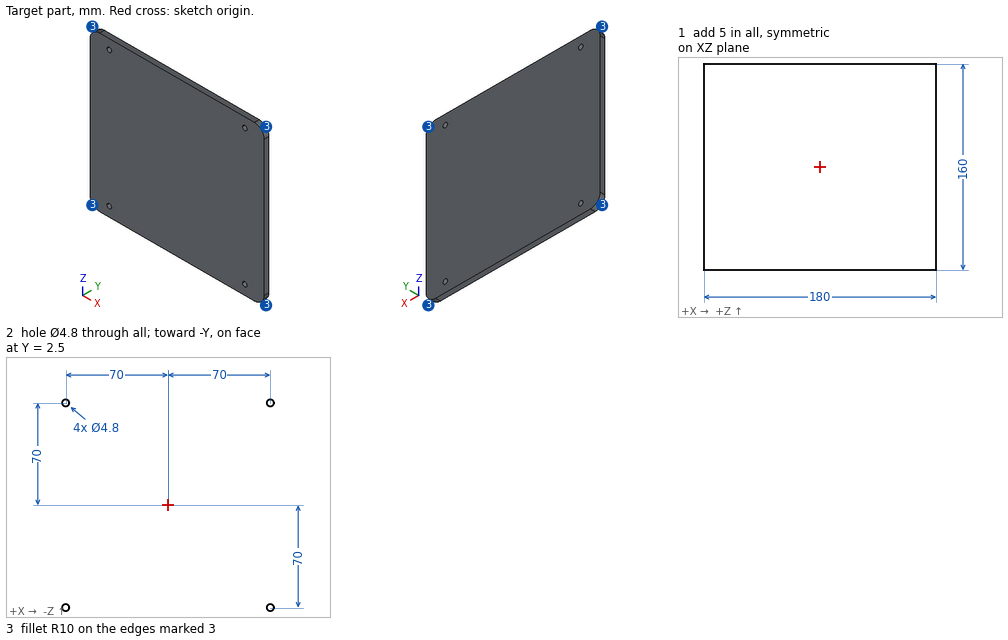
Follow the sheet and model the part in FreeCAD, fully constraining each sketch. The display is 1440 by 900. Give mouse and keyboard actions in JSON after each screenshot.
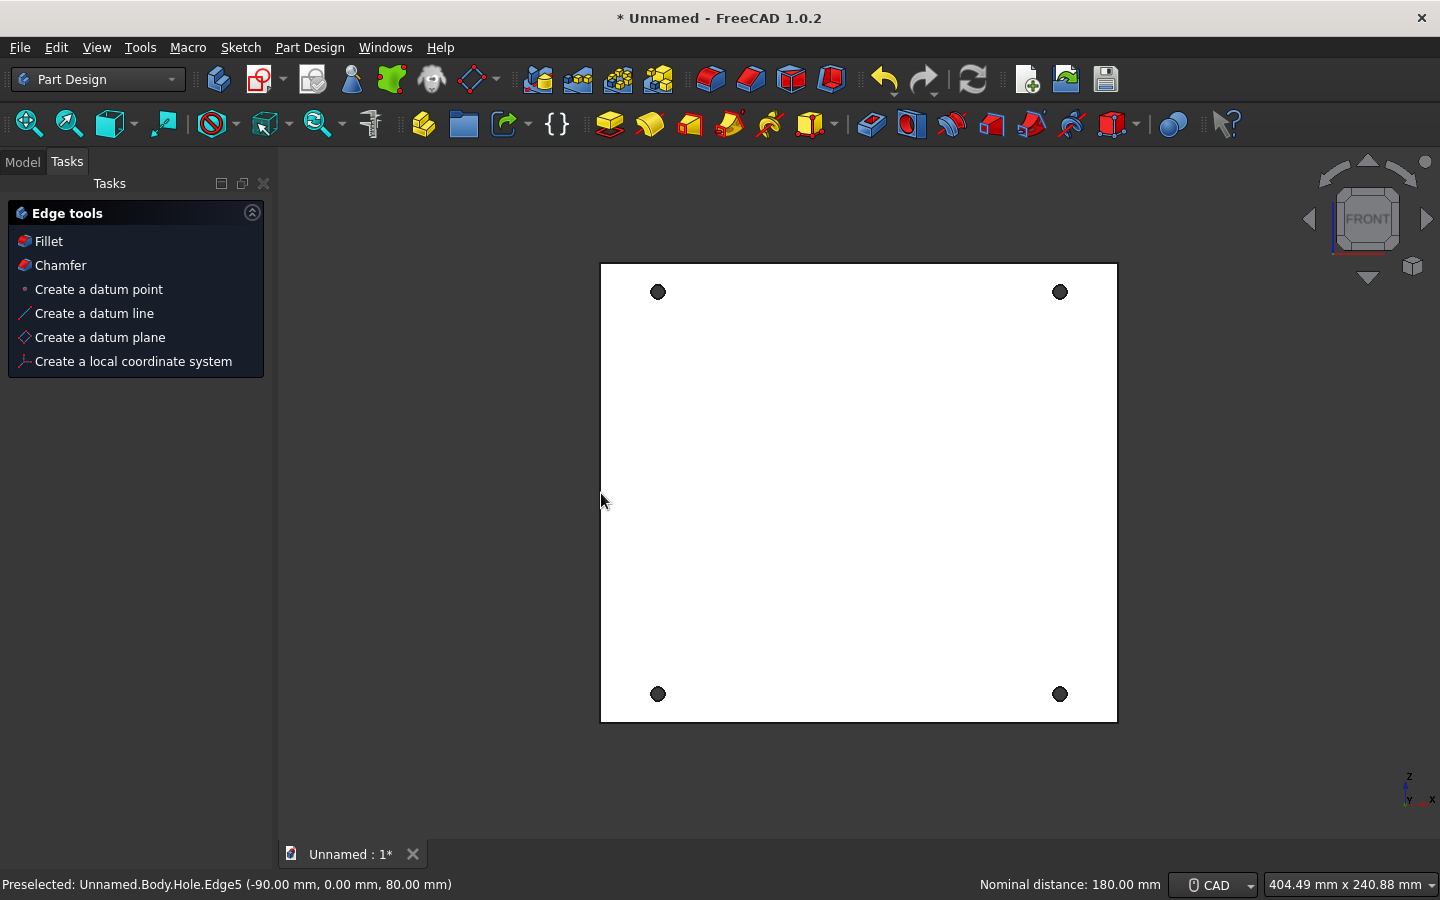
{"action": "scroll", "coordinate": [600, 722], "scroll_direction": "up", "scroll_amount": 6}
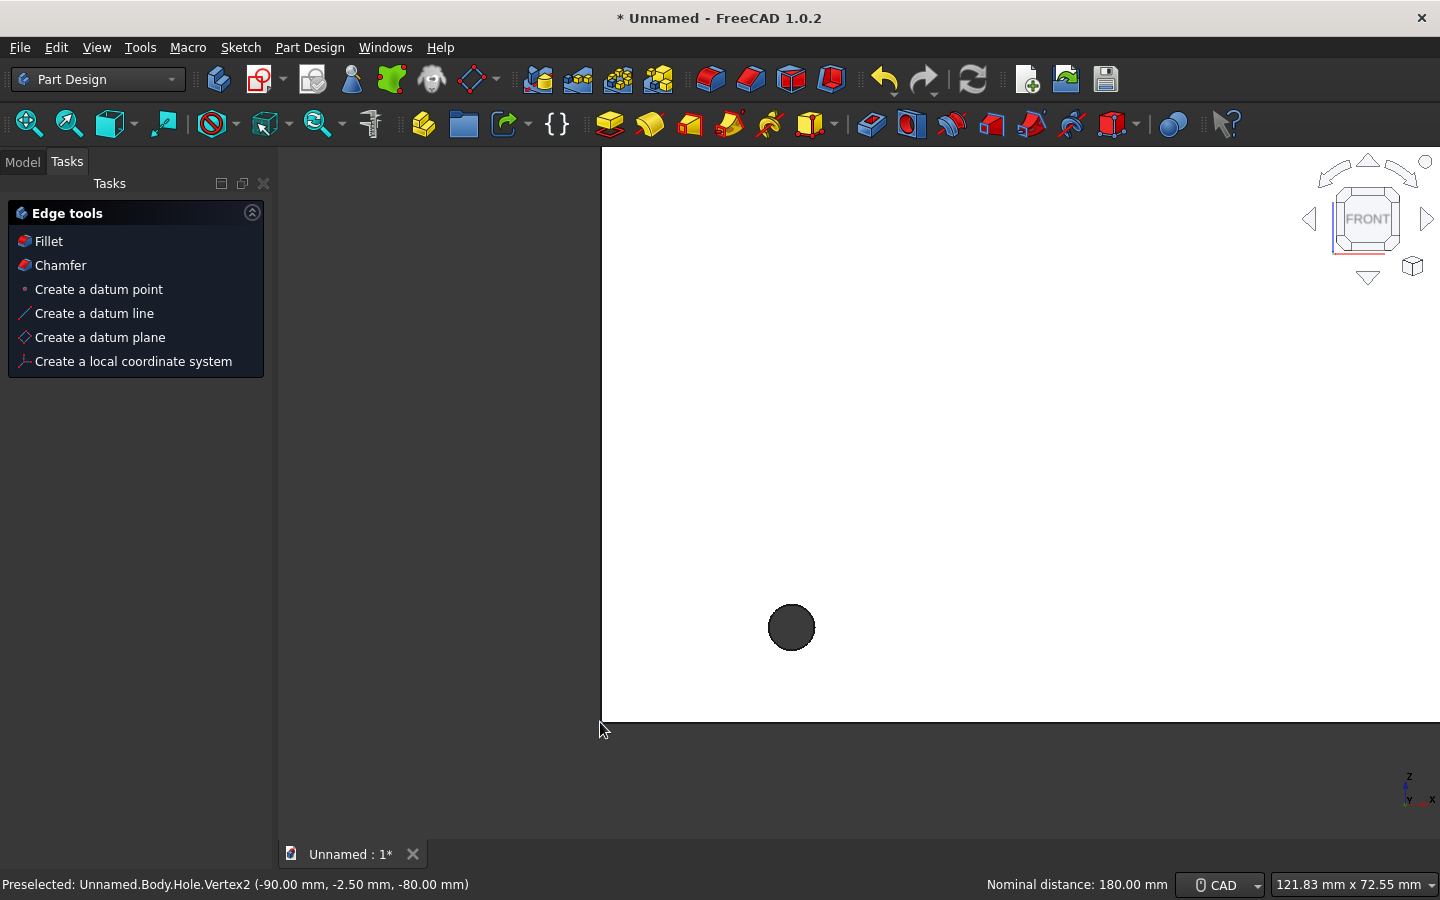
{"action": "left_click", "coordinate": [30, 124]}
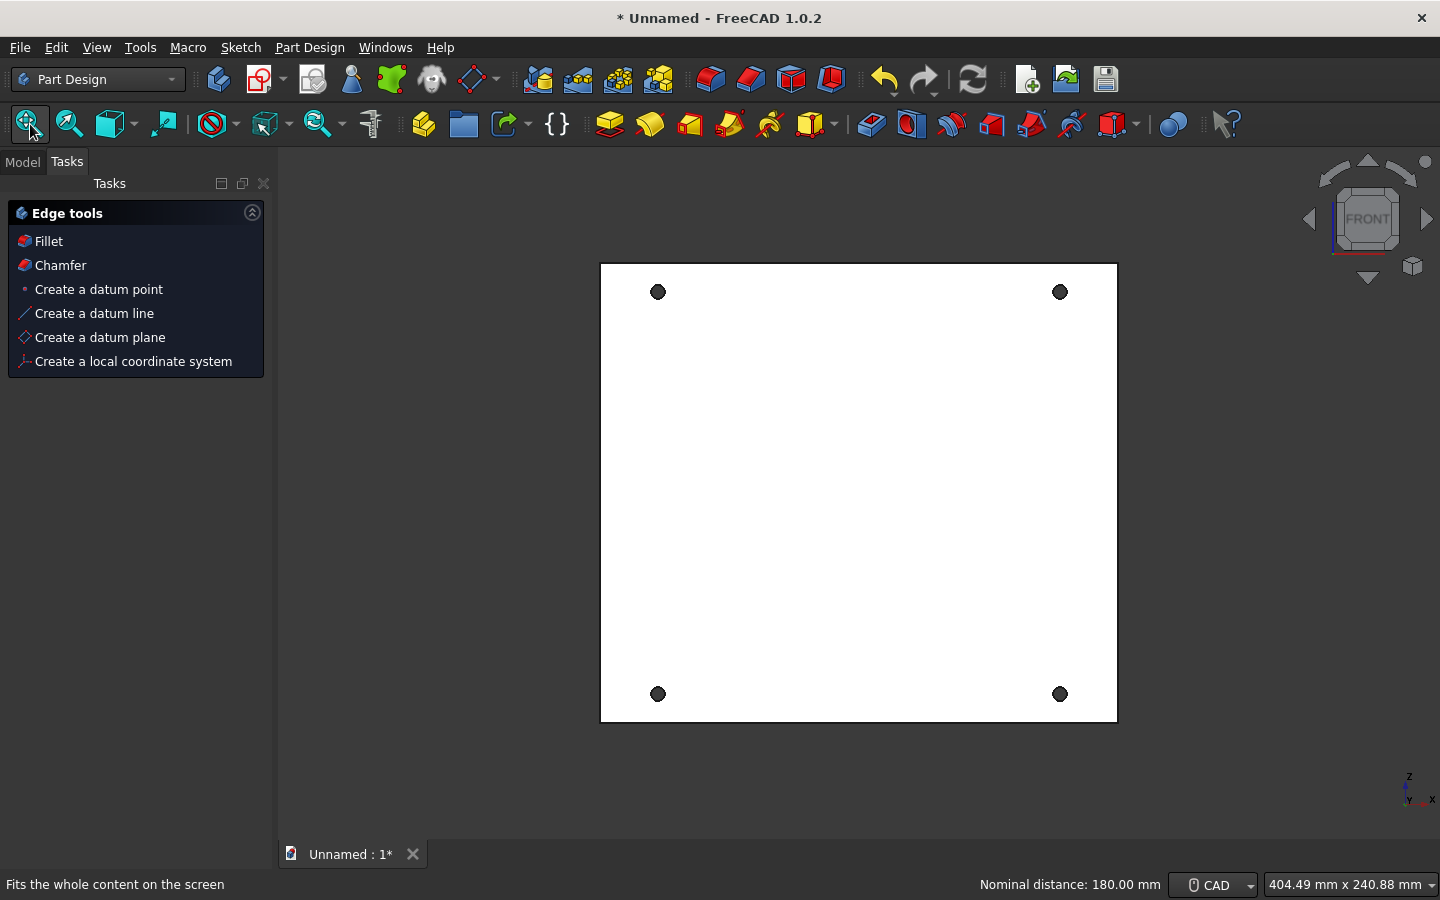
{"action": "key", "text": "3"}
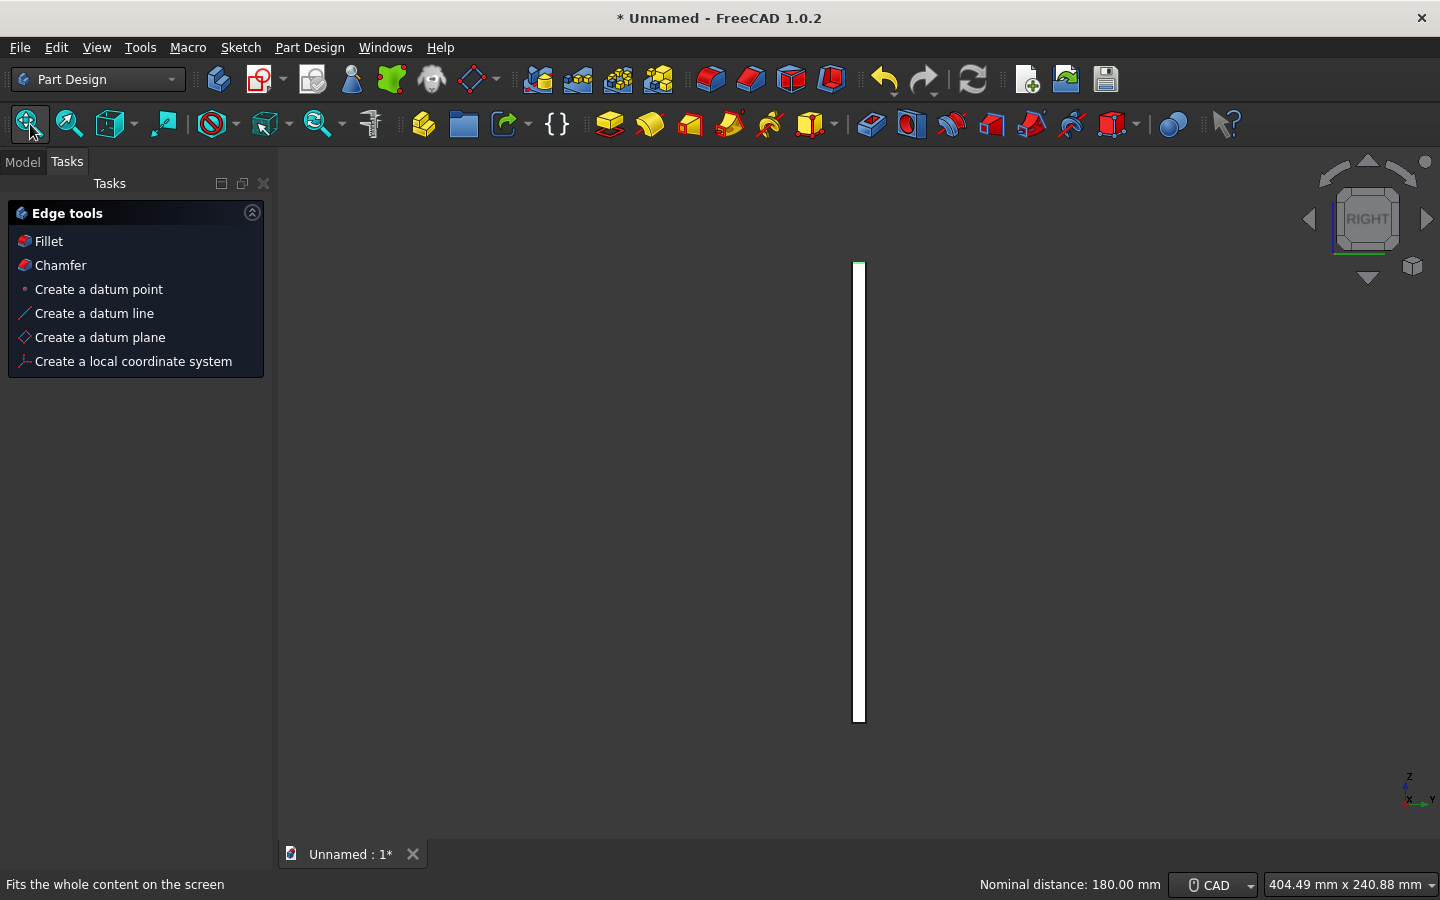
{"action": "left_click", "coordinate": [859, 722], "text": "ctrl"}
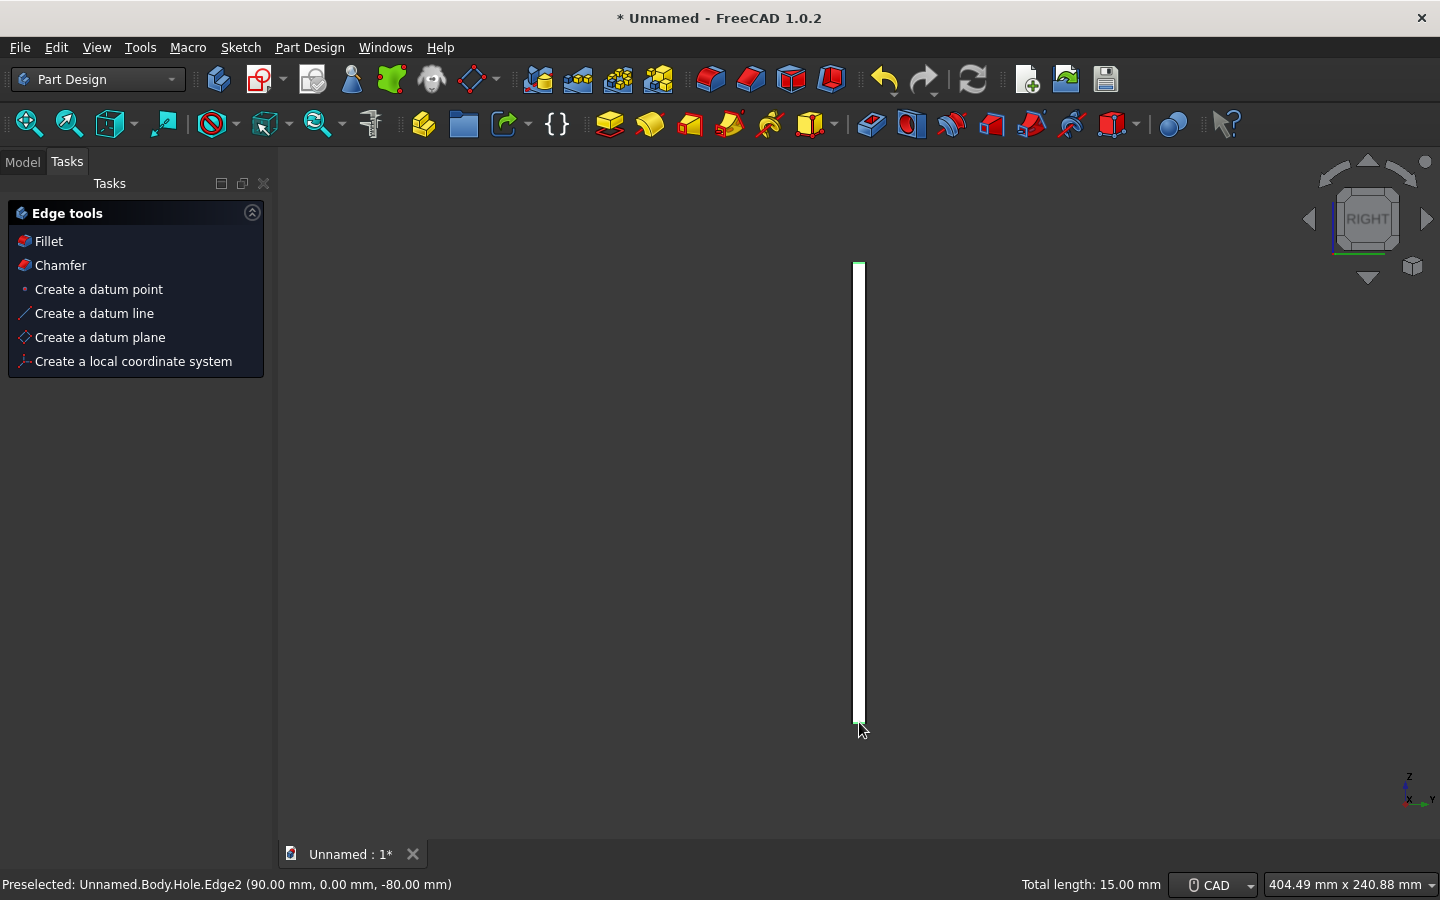
{"action": "scroll", "coordinate": [859, 722], "scroll_direction": "up", "scroll_amount": 6}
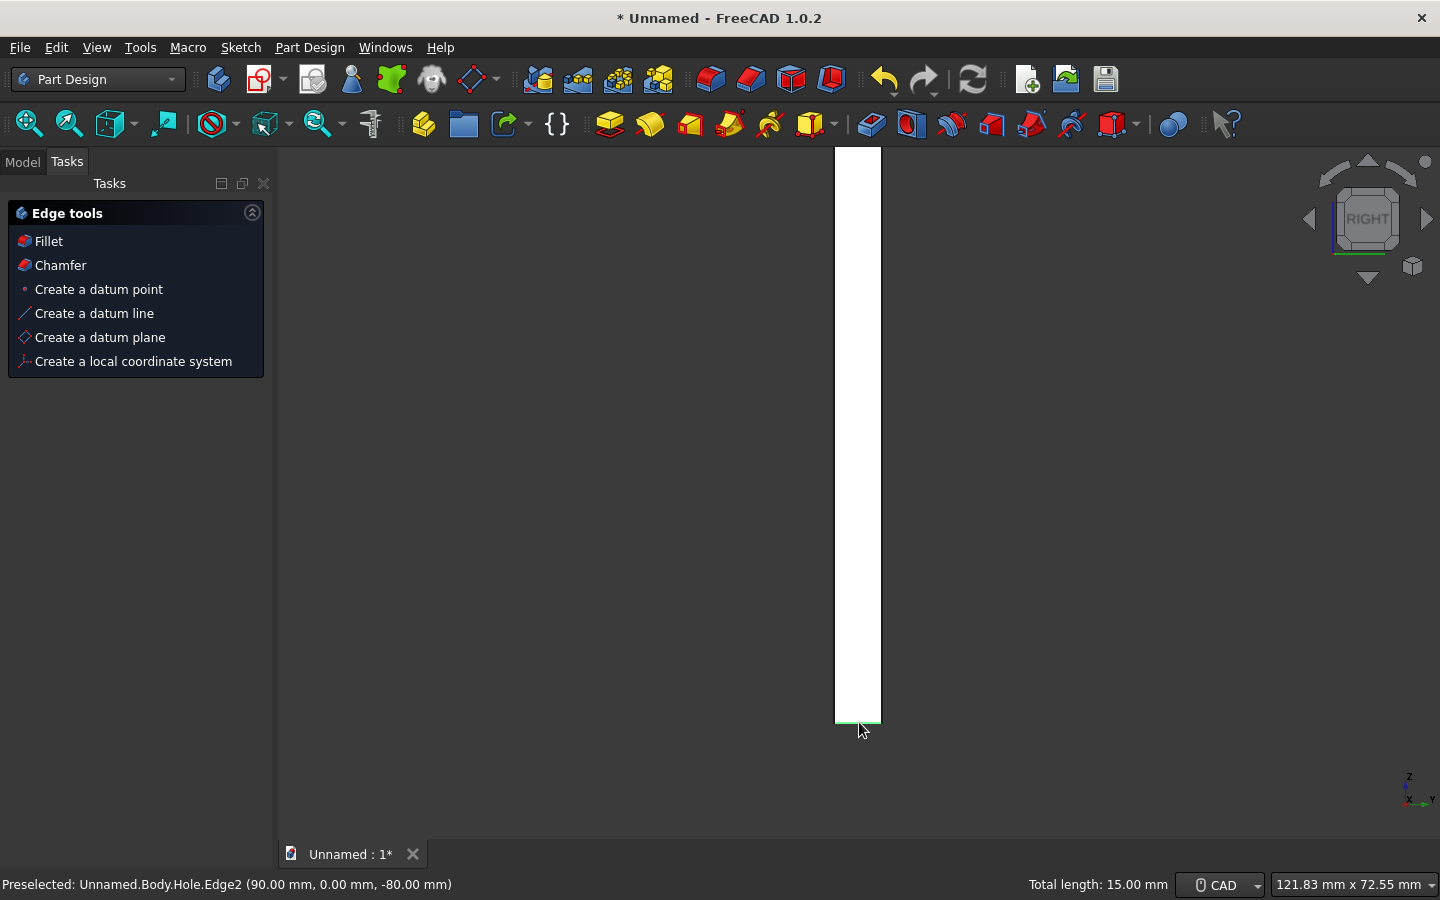
{"action": "left_click", "coordinate": [30, 124]}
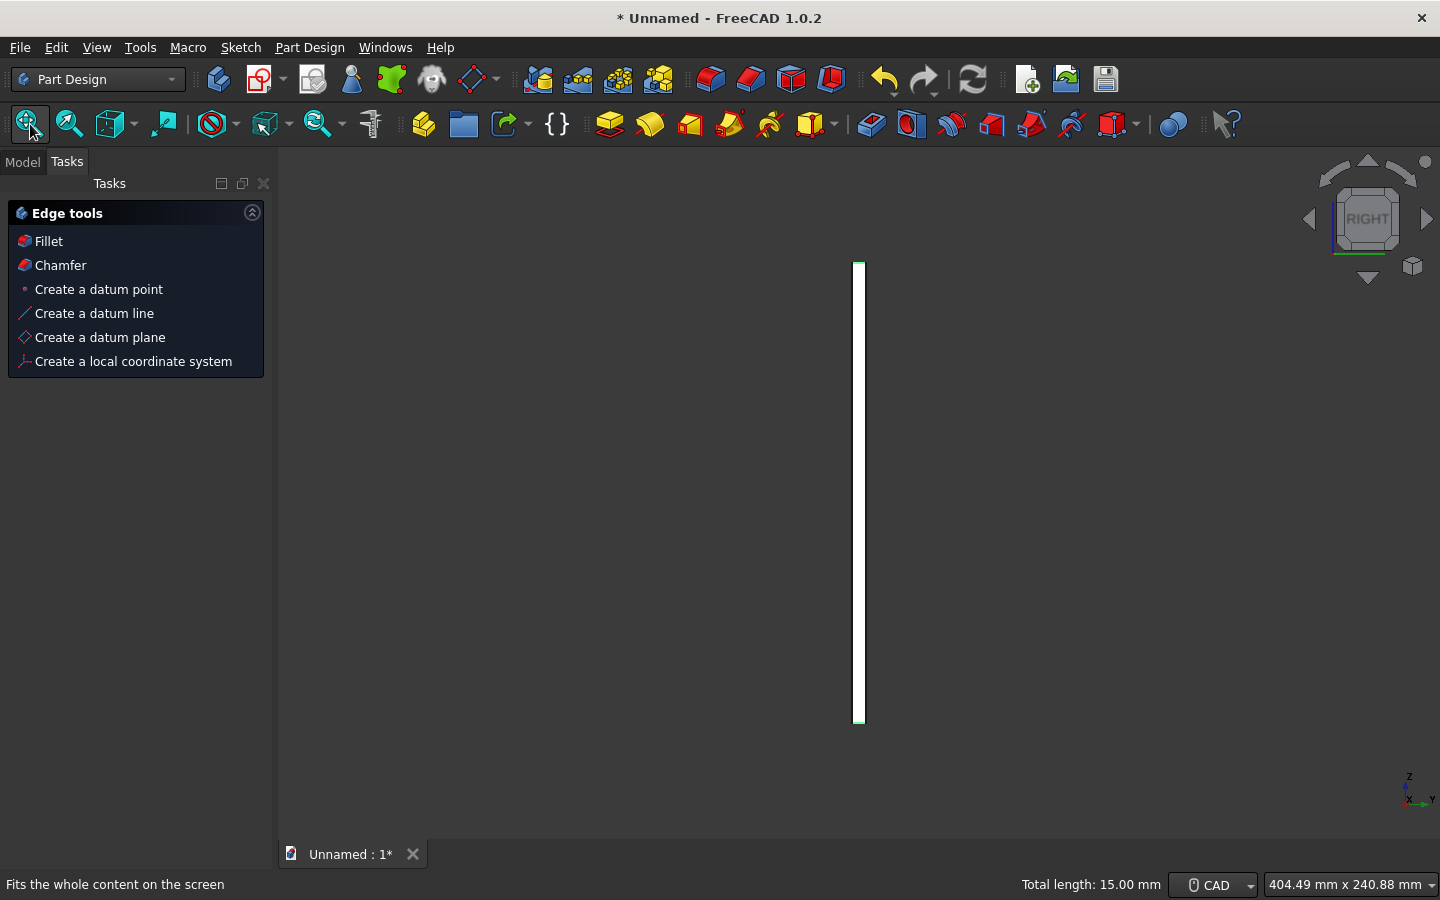
{"action": "key", "text": "5"}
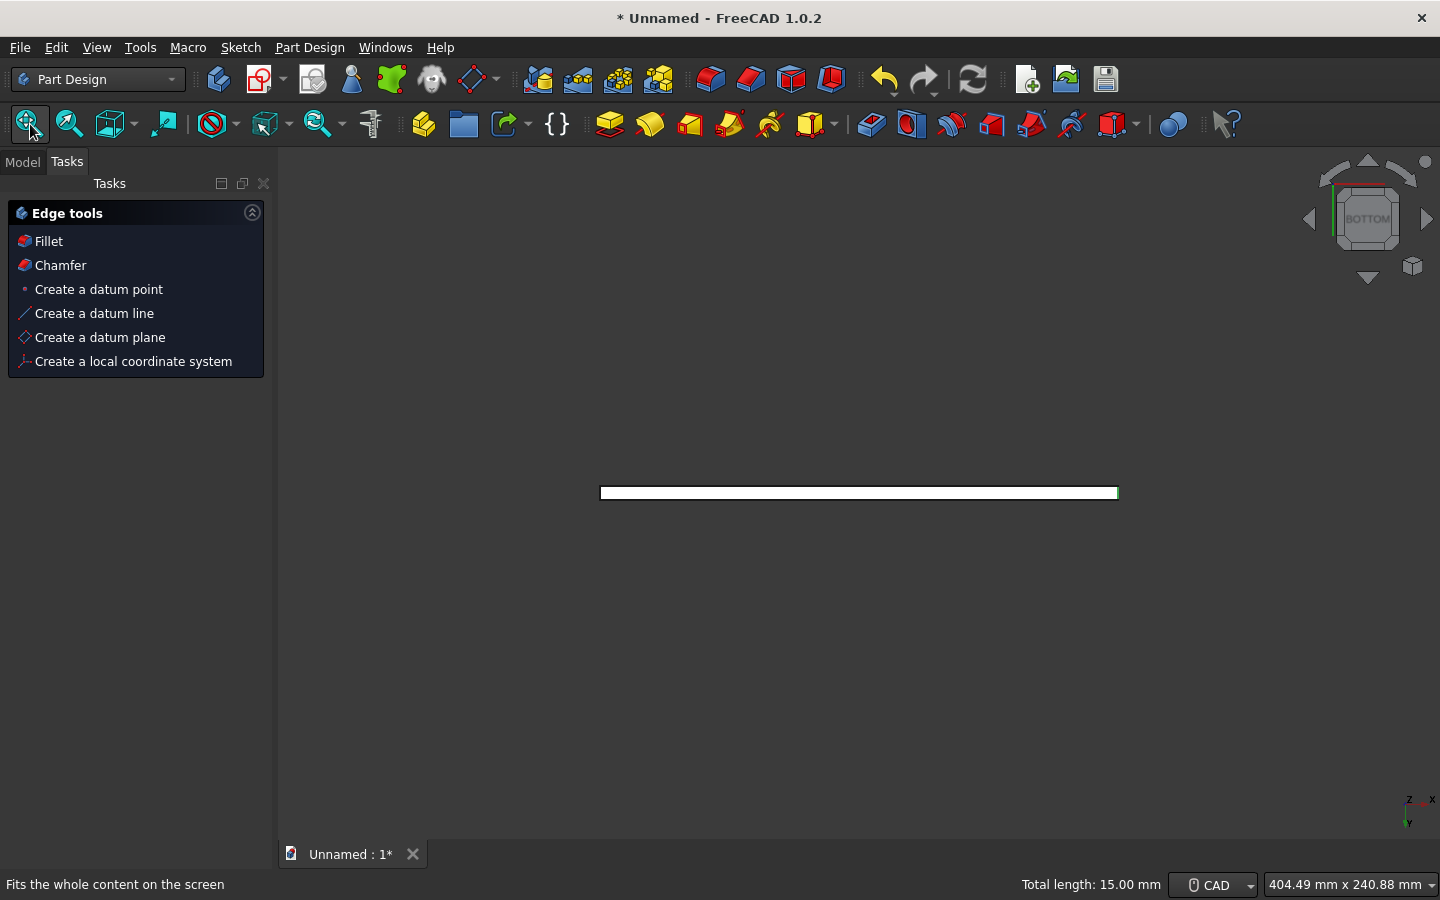
{"action": "key", "text": "v f"}